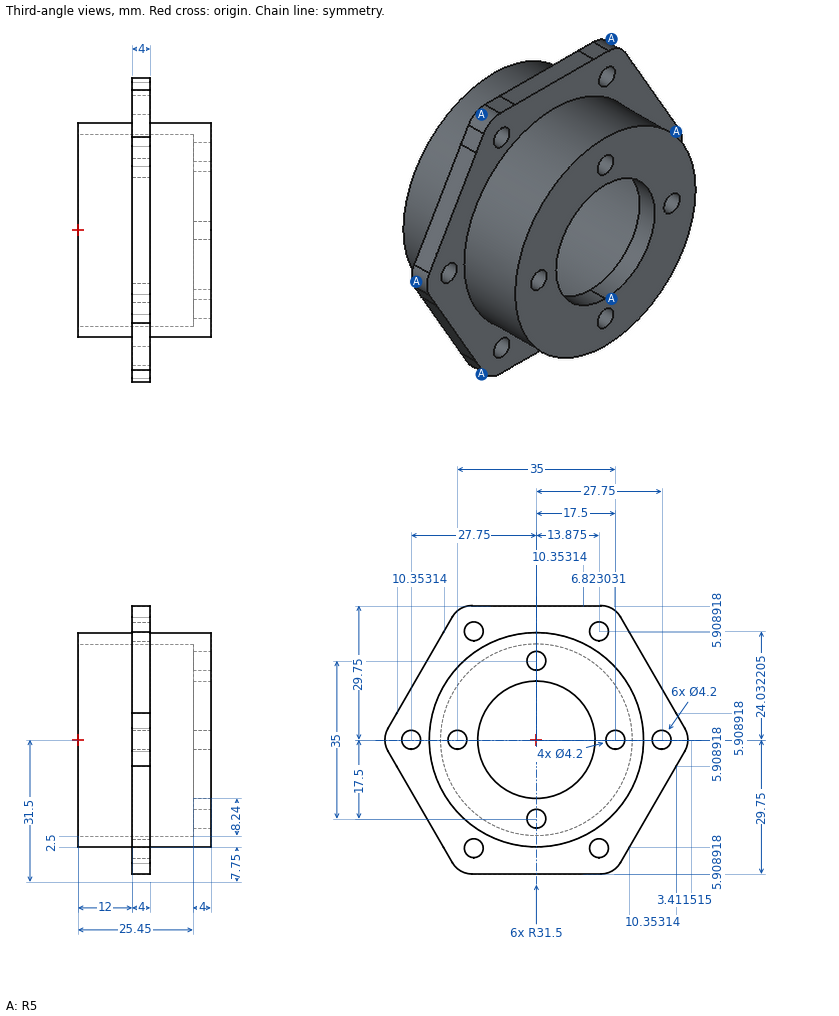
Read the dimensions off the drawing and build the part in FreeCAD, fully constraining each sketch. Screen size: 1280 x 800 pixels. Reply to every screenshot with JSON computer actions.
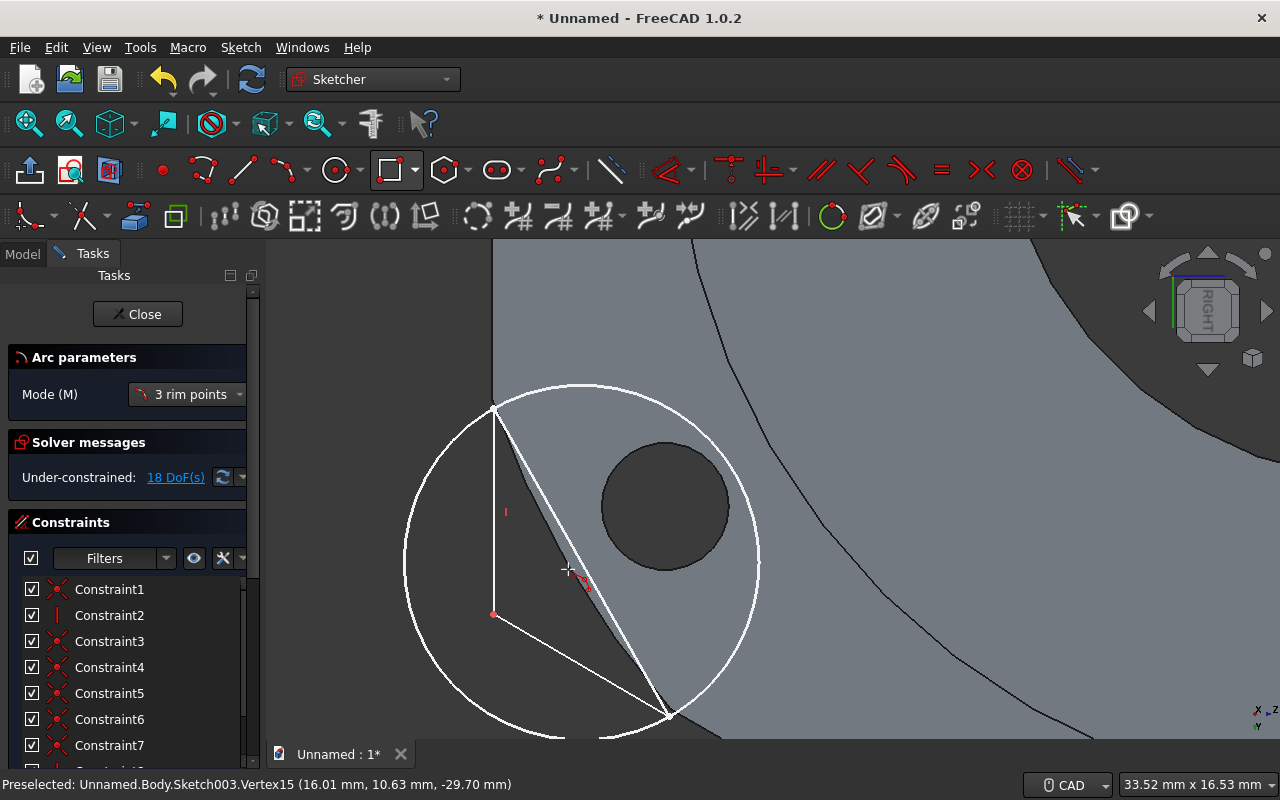
{"action": "left_click", "coordinate": [567, 563]}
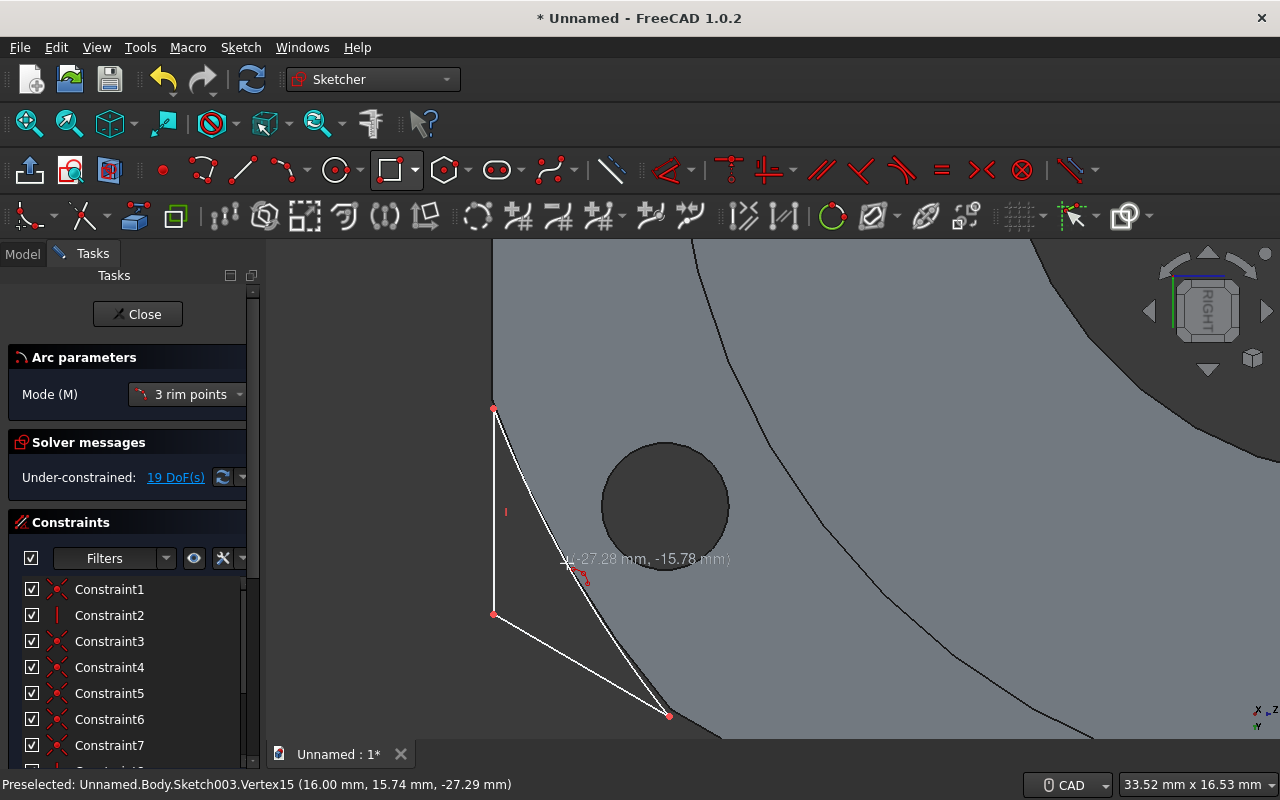
{"action": "left_click", "coordinate": [204, 170]}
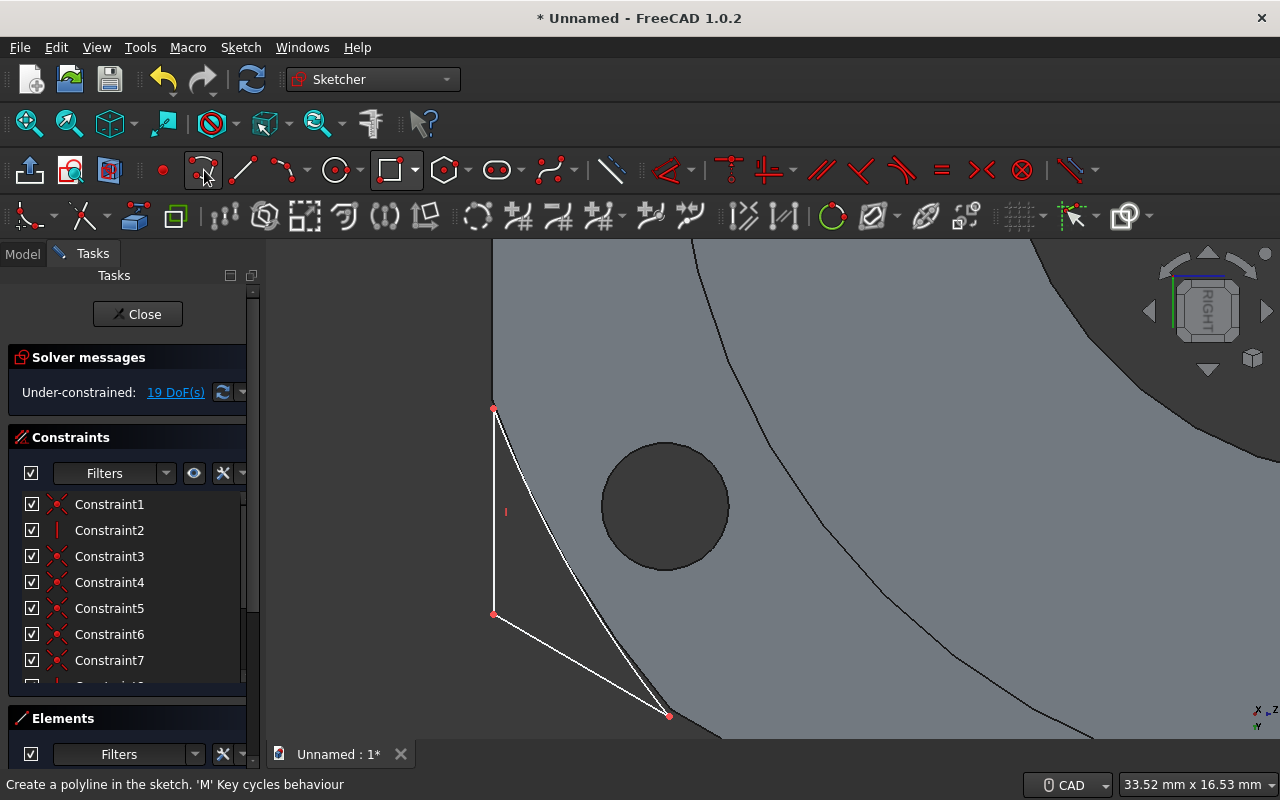
{"action": "scroll", "coordinate": [568, 569], "scroll_direction": "down", "scroll_amount": 9}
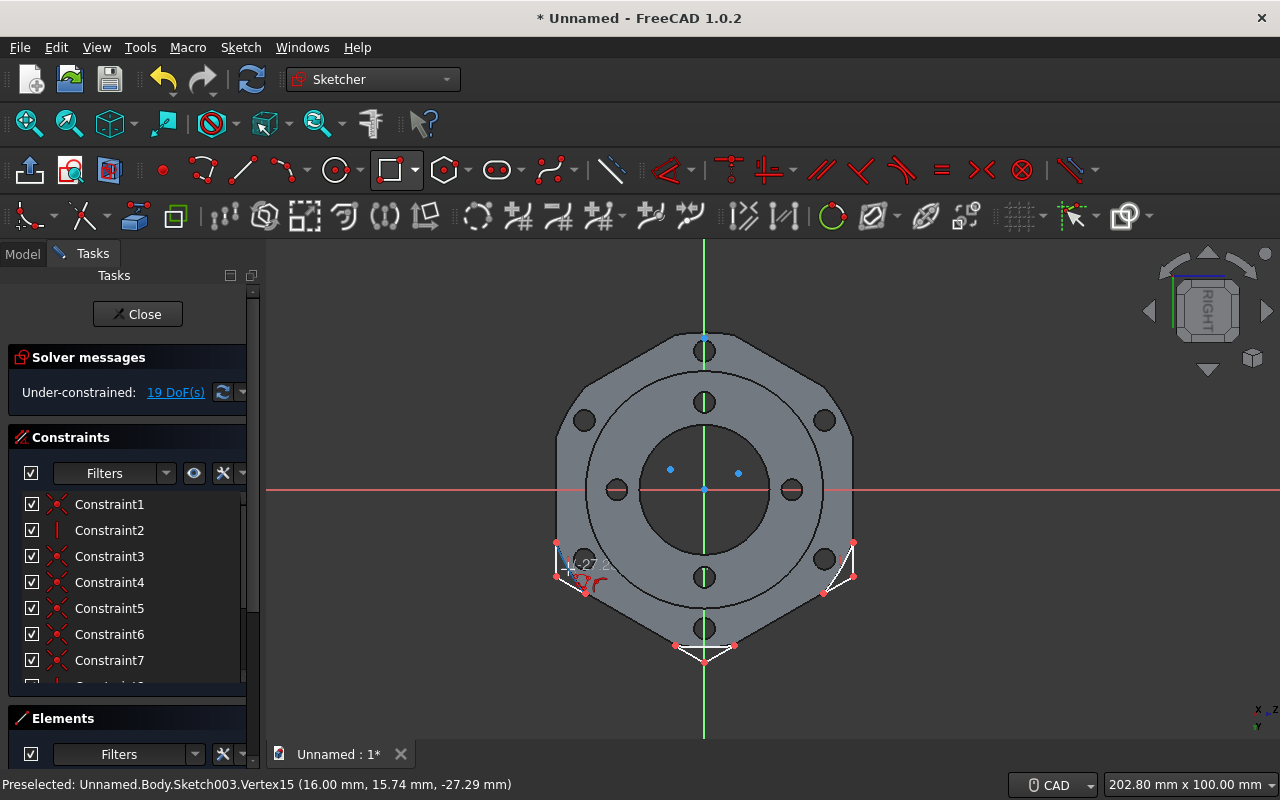
{"action": "left_click", "coordinate": [585, 387]}
{"action": "left_click", "coordinate": [556, 404]}
{"action": "left_click", "coordinate": [556, 438]}
{"action": "right_click", "coordinate": [556, 438]}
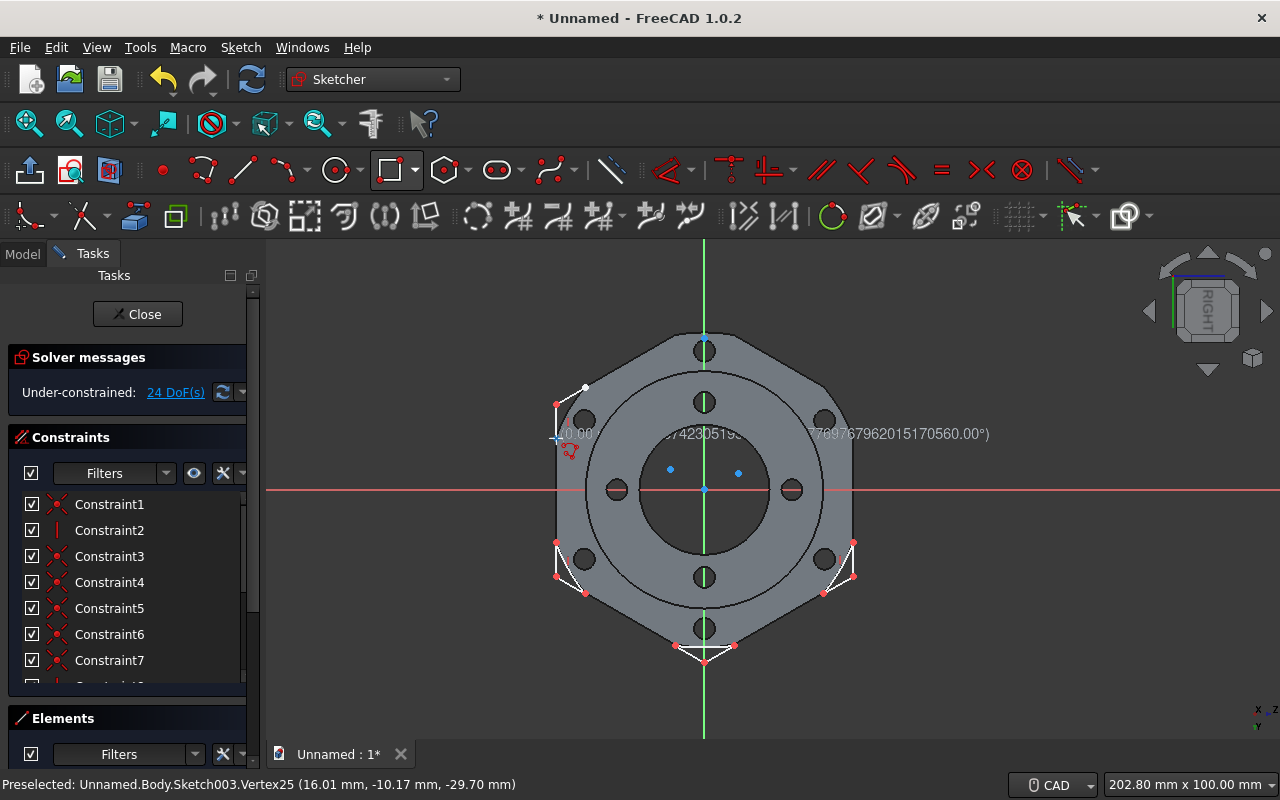
{"action": "key", "text": "g 3 a"}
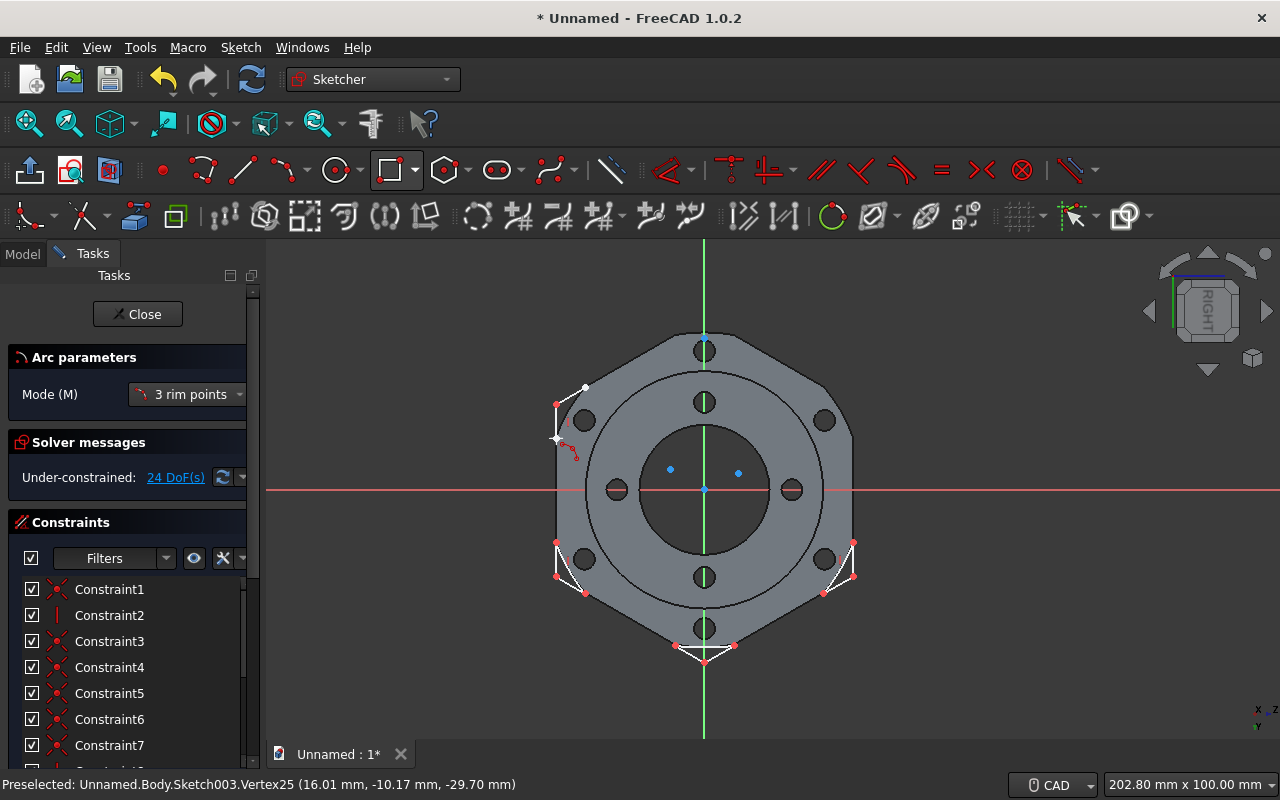
{"action": "left_click", "coordinate": [556, 439]}
{"action": "left_click", "coordinate": [585, 388]}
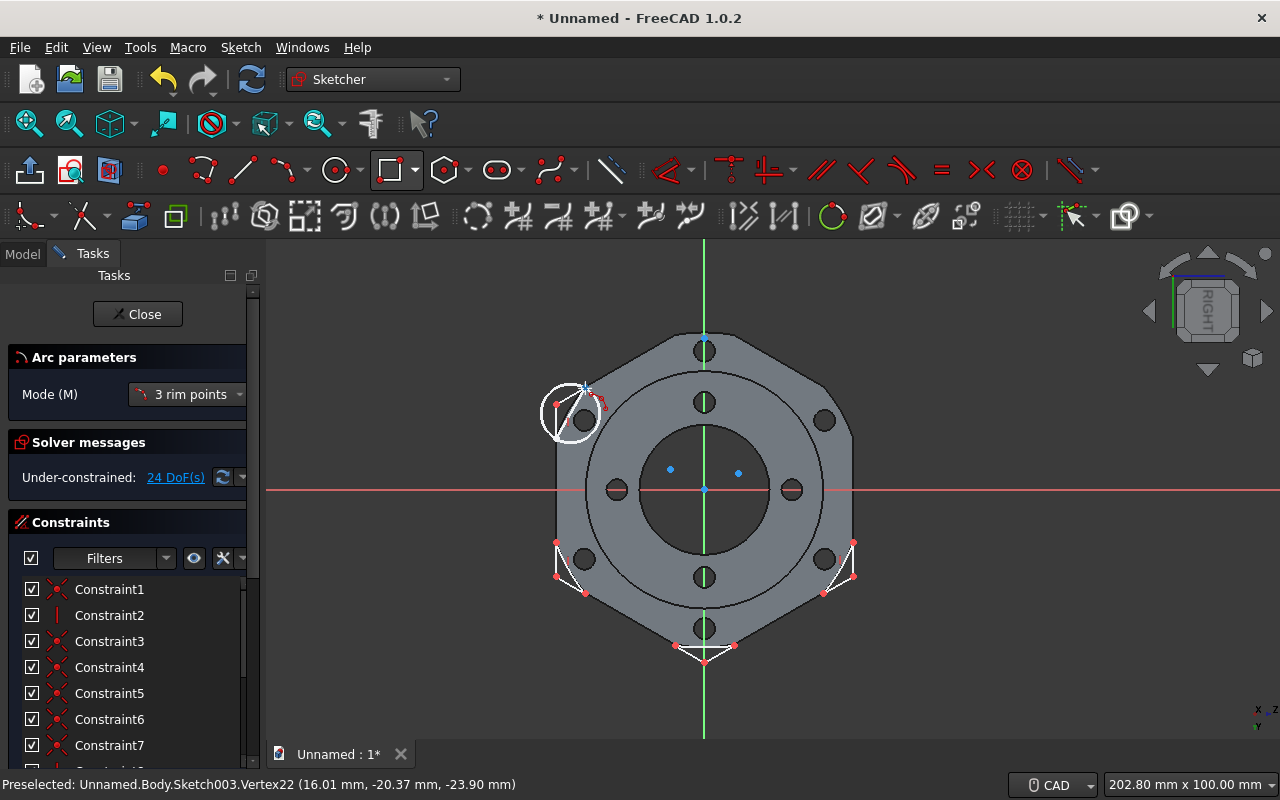
{"action": "scroll", "coordinate": [568, 411], "scroll_direction": "up", "scroll_amount": 9}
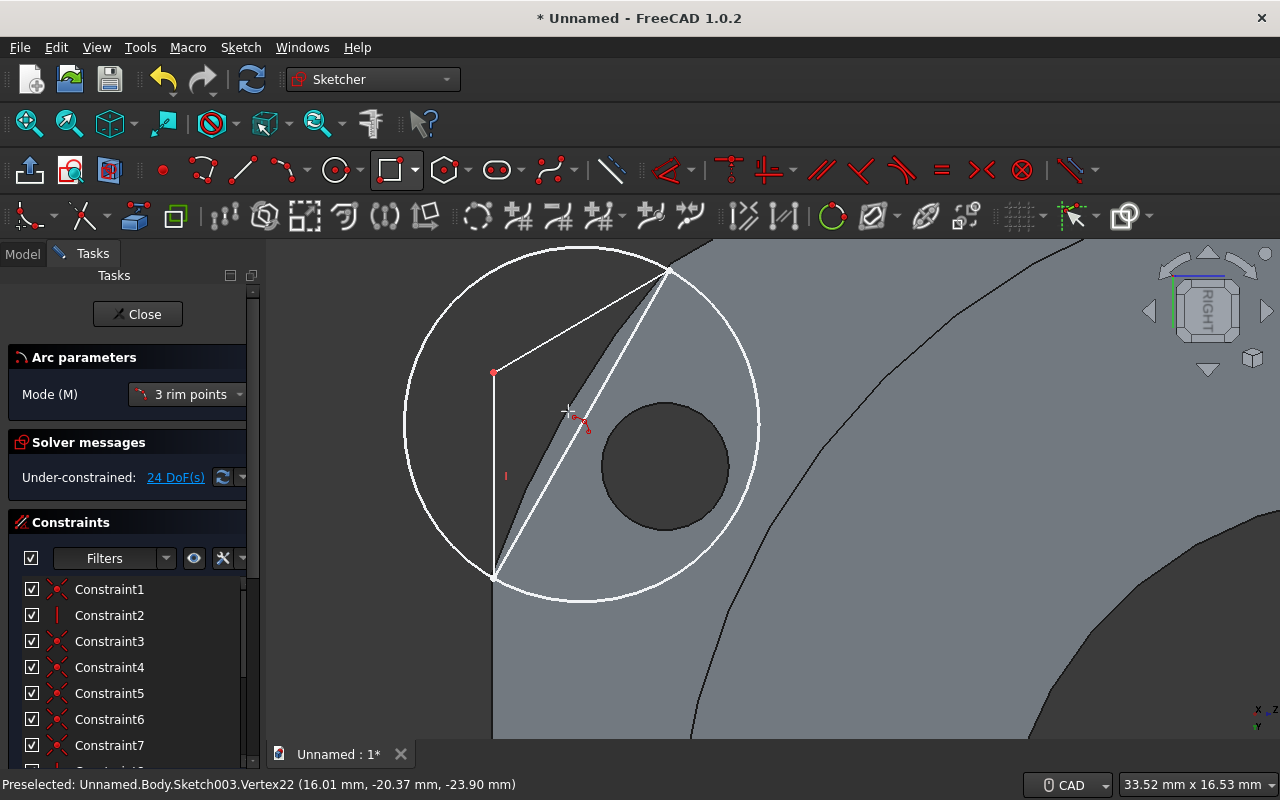
{"action": "left_click", "coordinate": [567, 410]}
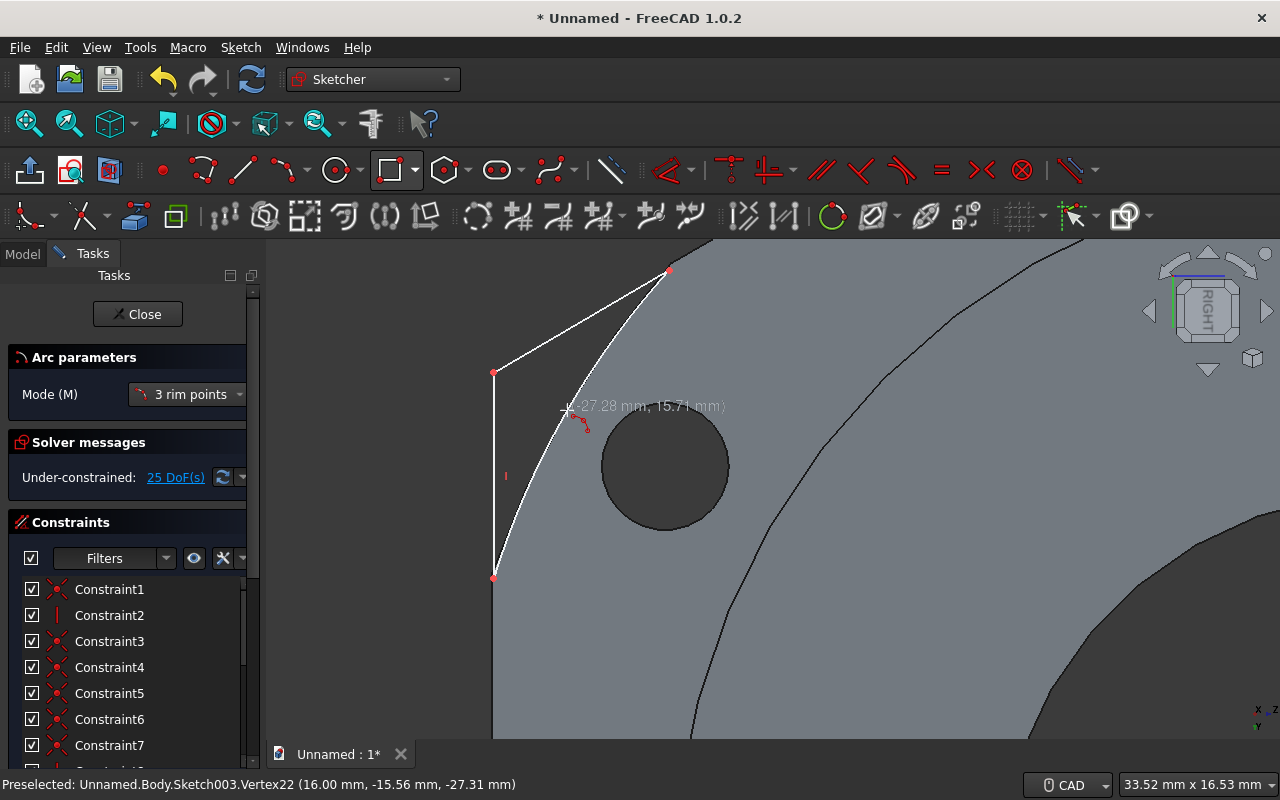
{"action": "left_click", "coordinate": [204, 170]}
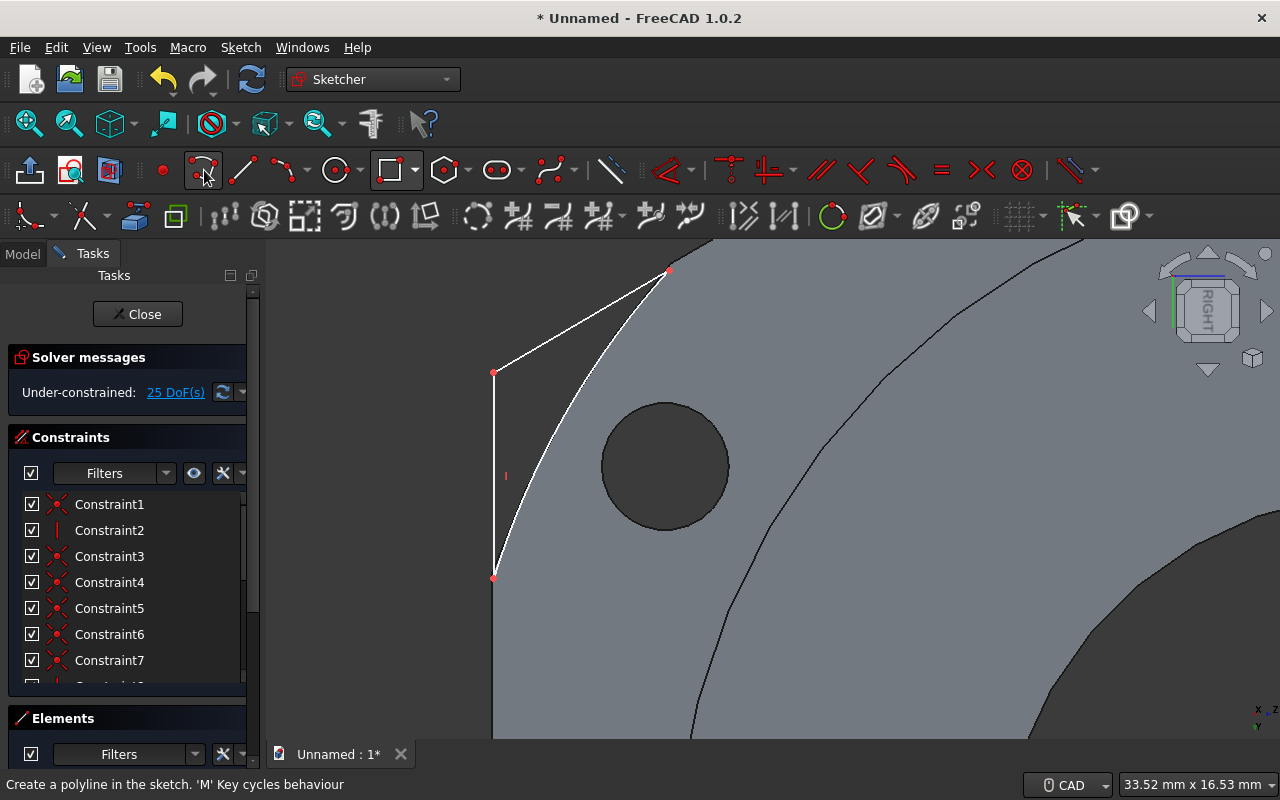
{"action": "scroll", "coordinate": [568, 410], "scroll_direction": "down", "scroll_amount": 9}